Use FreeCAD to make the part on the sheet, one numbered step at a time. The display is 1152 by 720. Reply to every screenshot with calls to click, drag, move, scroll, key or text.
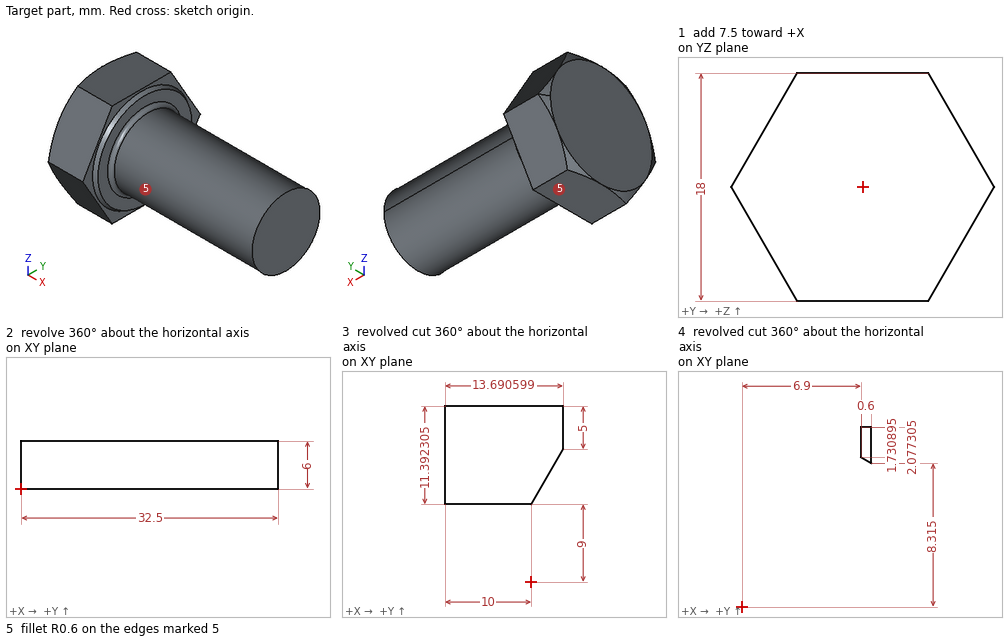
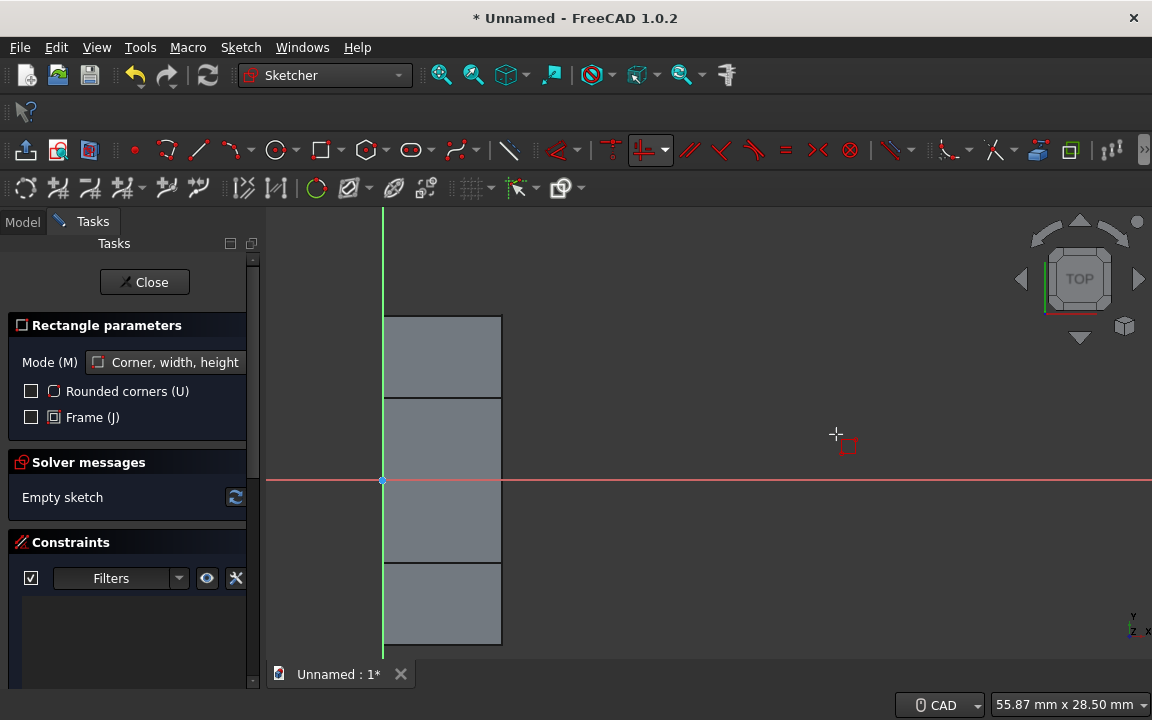
click(383, 480)
click(898, 385)
key(Escape)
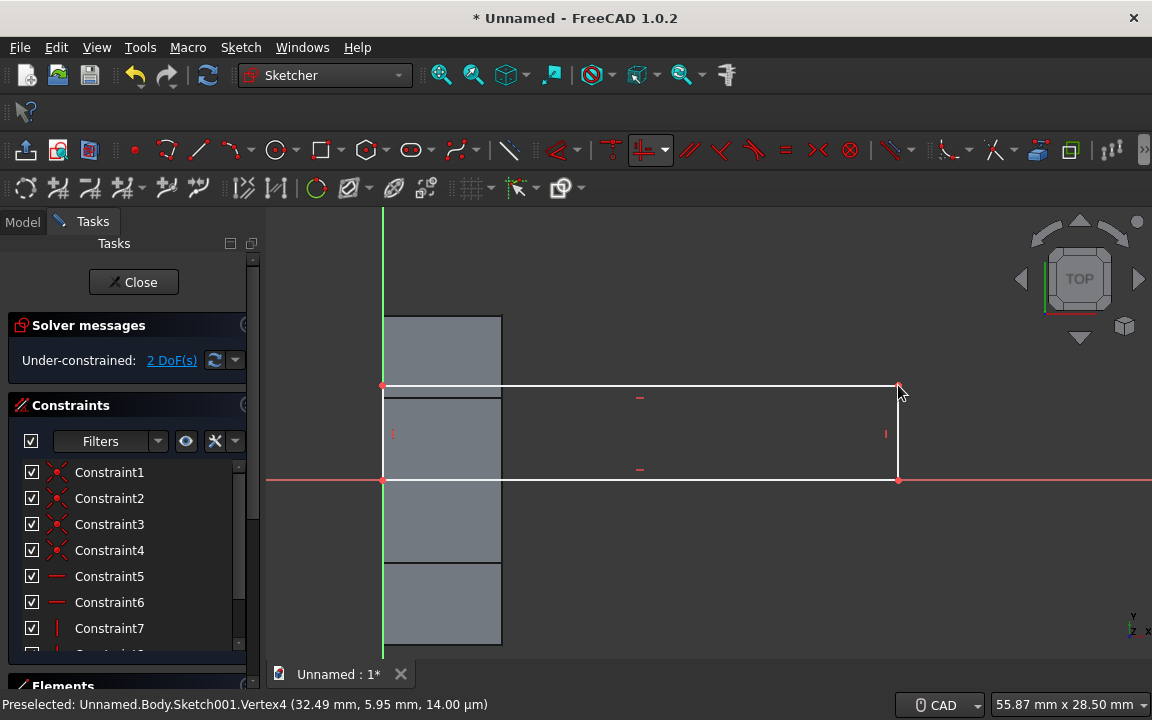
click(898, 452)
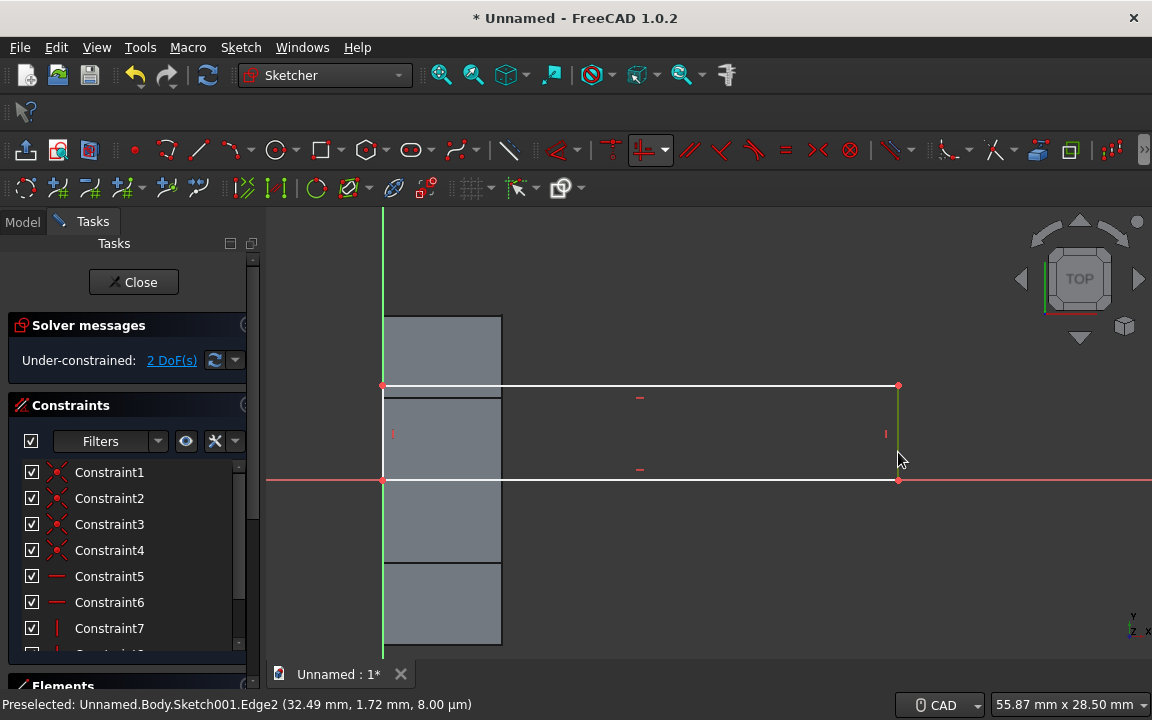
click(580, 150)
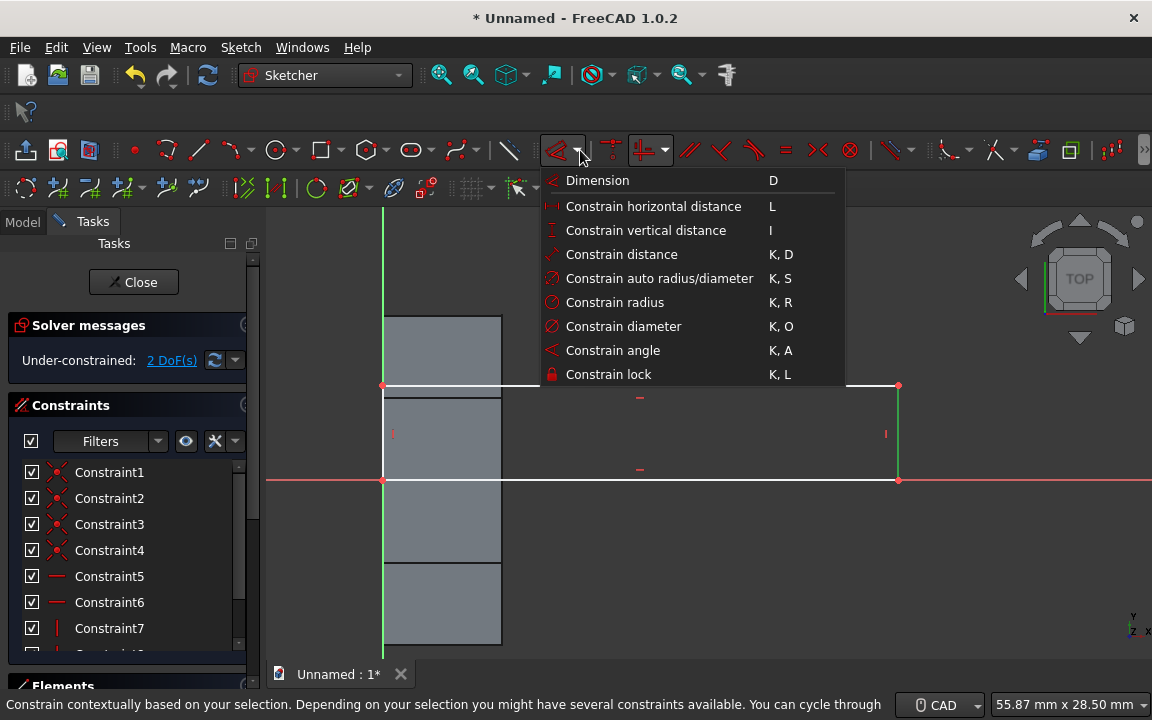
click(693, 230)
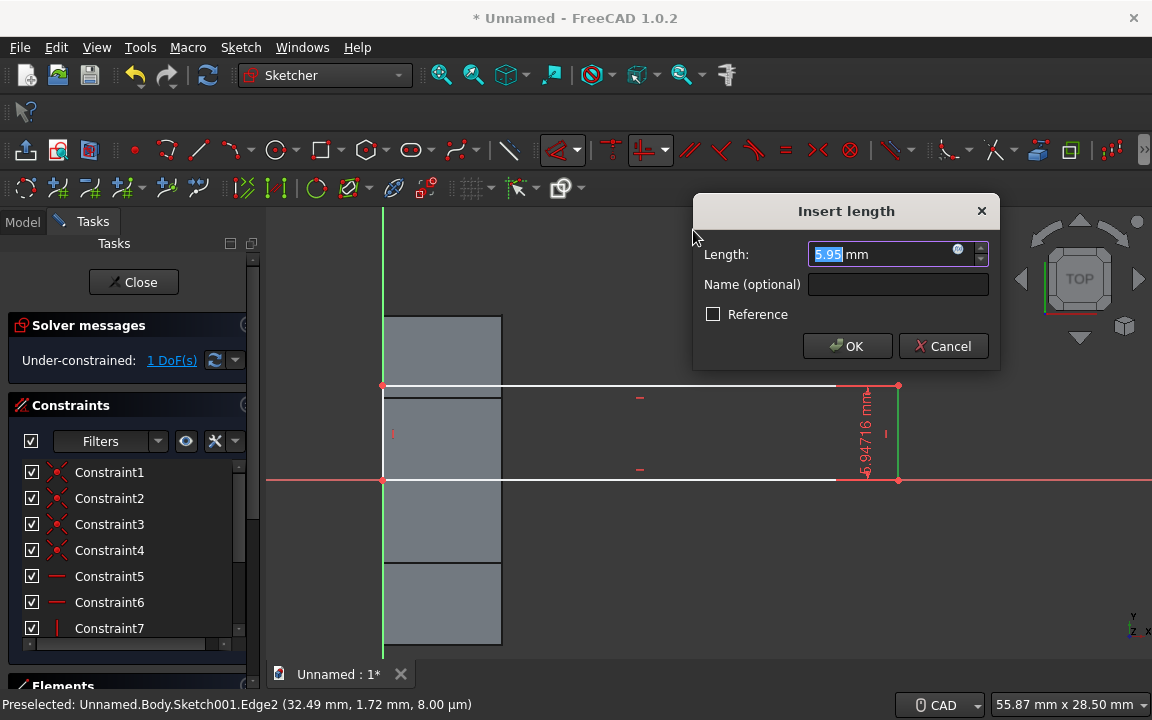
text(6)
key(Return)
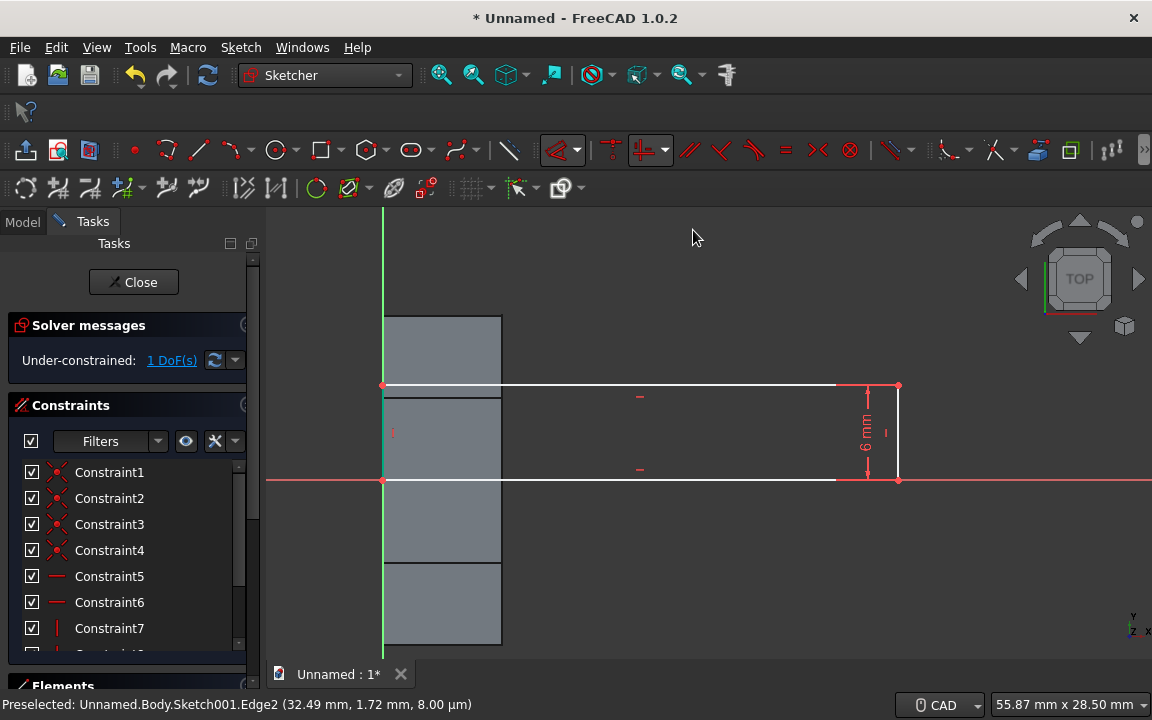
click(537, 480)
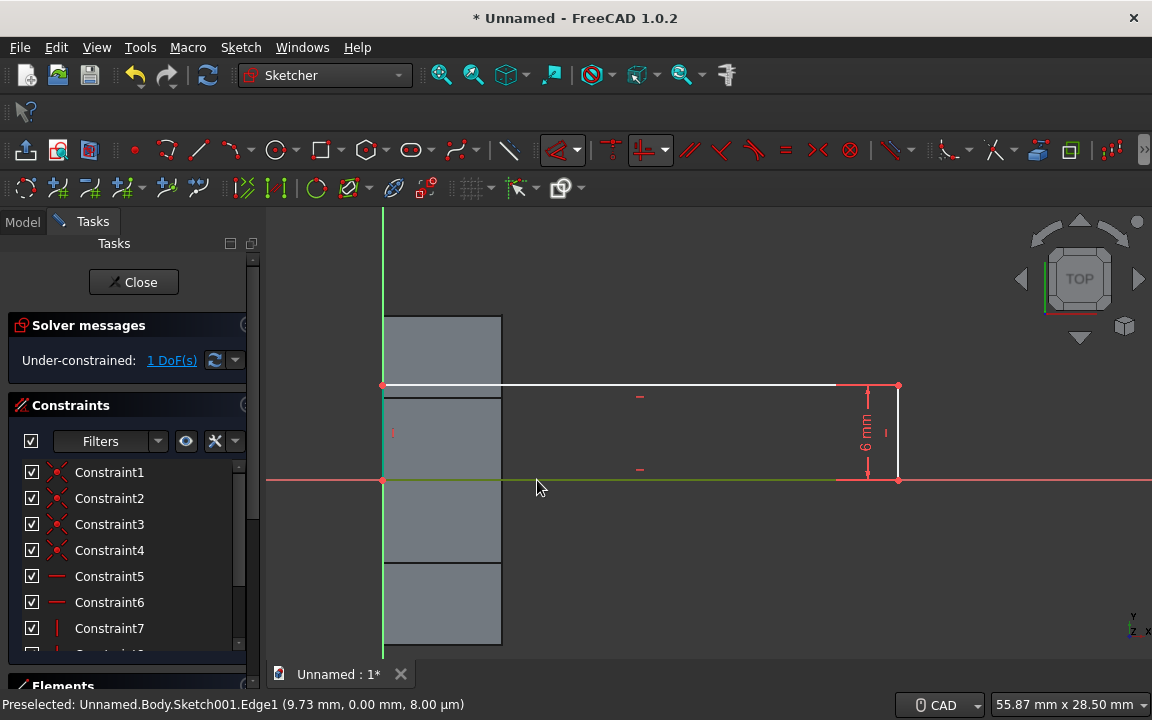
click(580, 150)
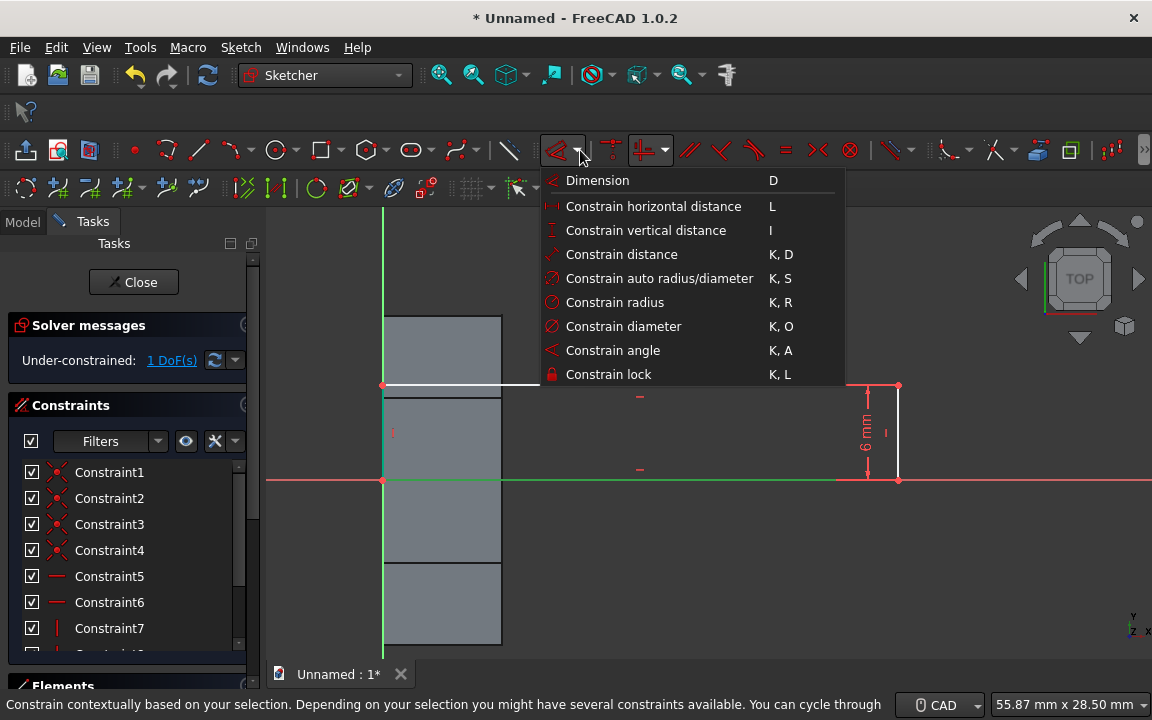
click(693, 206)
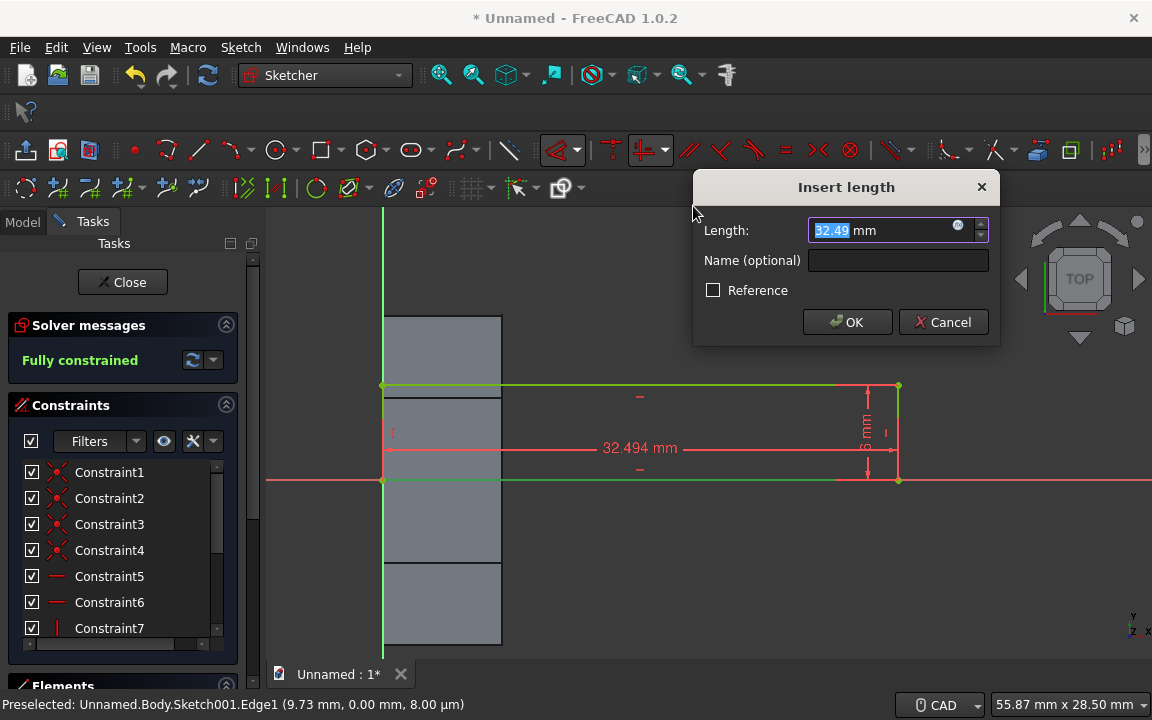
text(32.5)
key(Return)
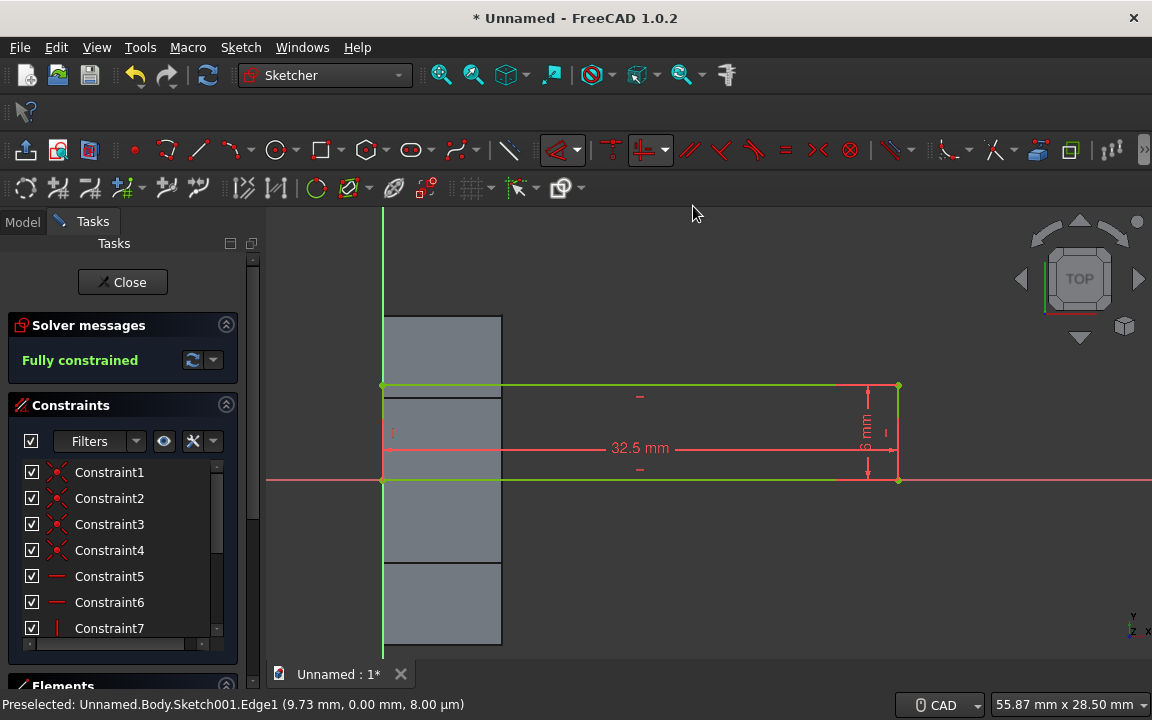
click(123, 282)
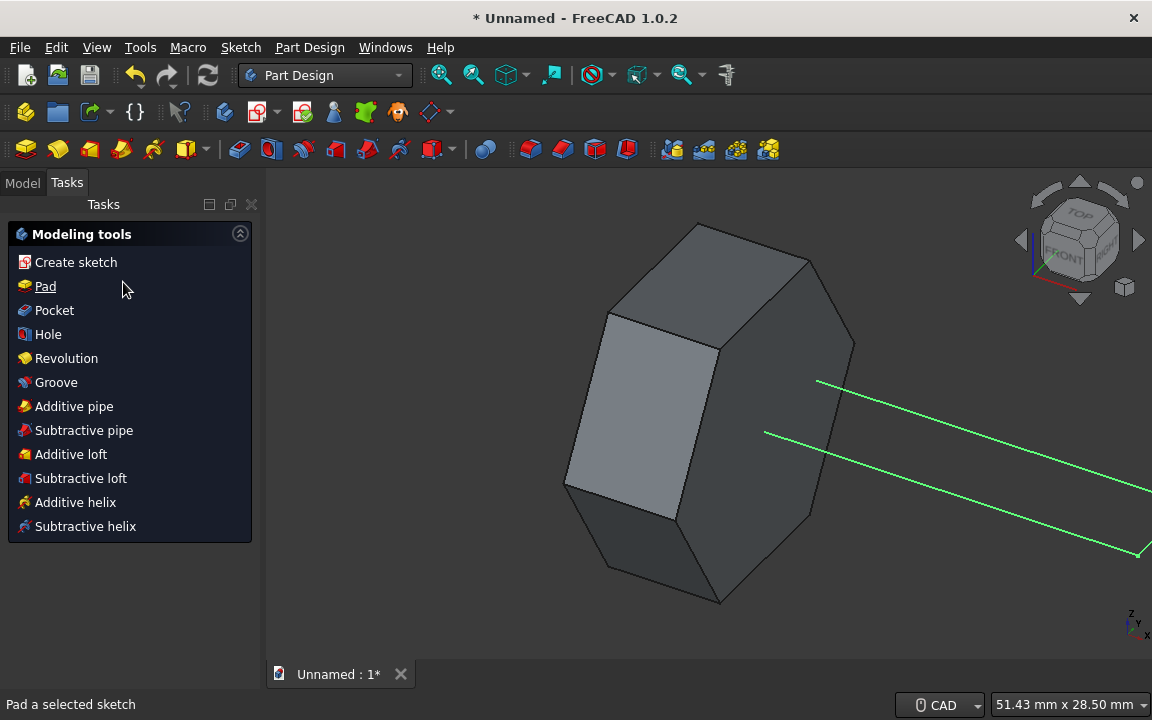
click(58, 150)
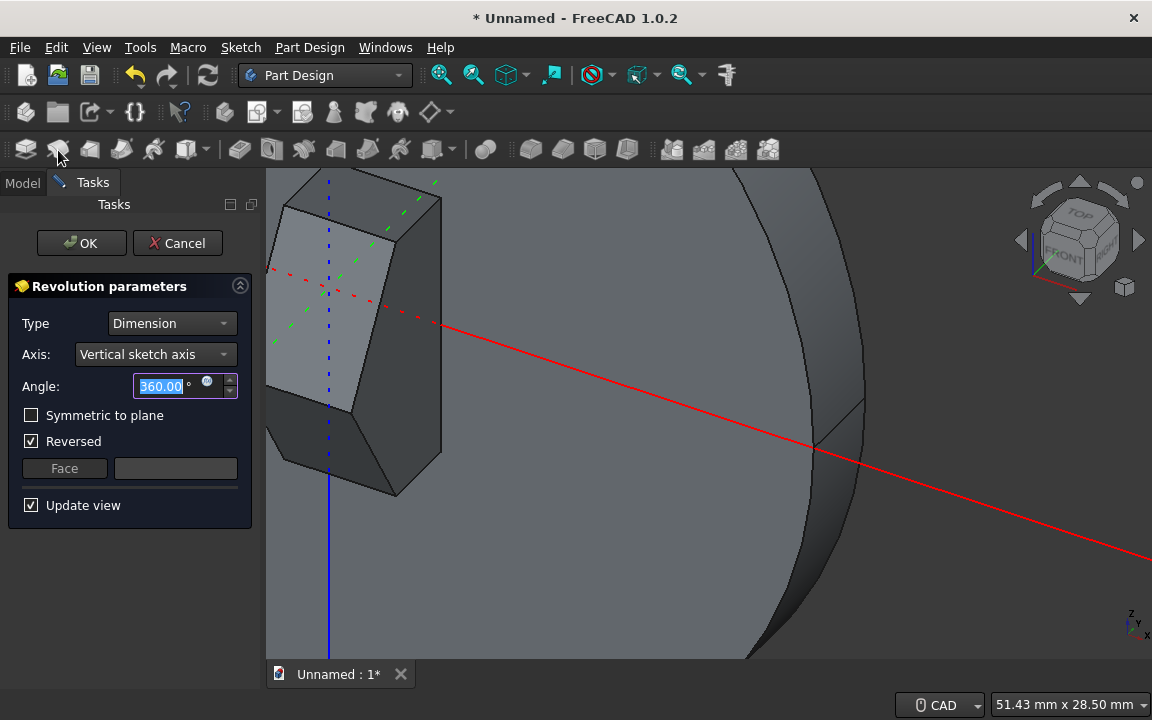
click(156, 354)